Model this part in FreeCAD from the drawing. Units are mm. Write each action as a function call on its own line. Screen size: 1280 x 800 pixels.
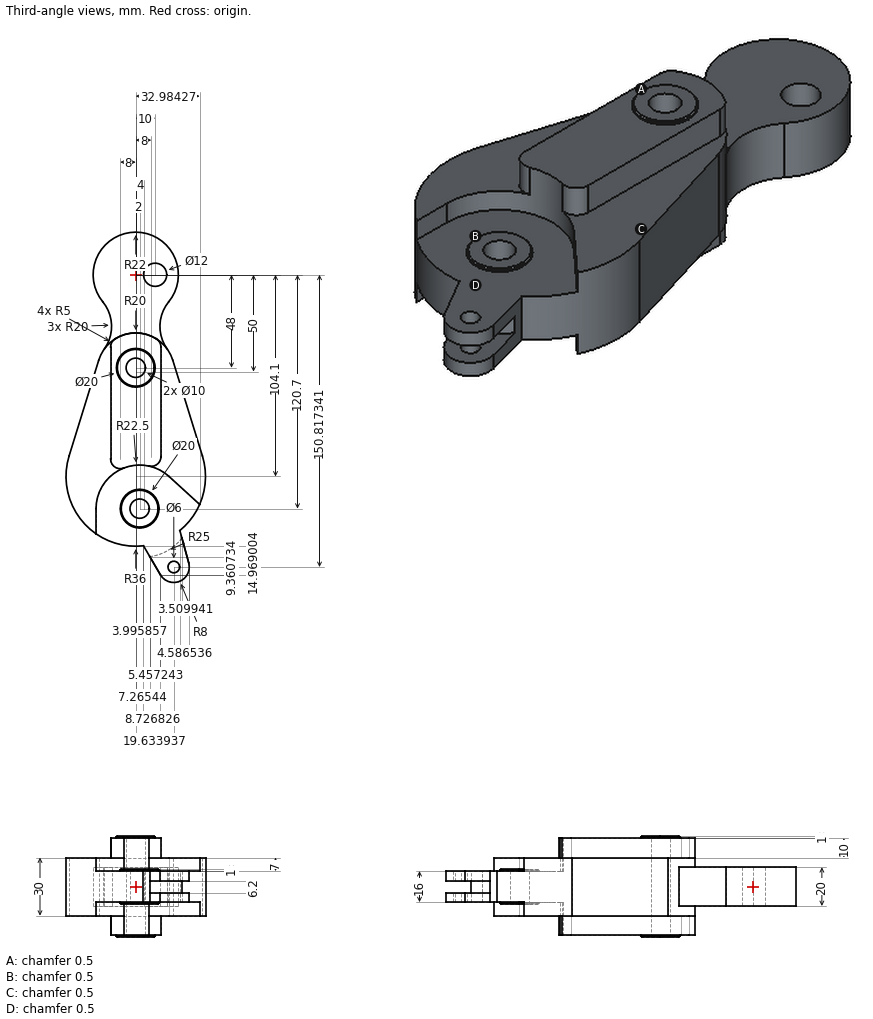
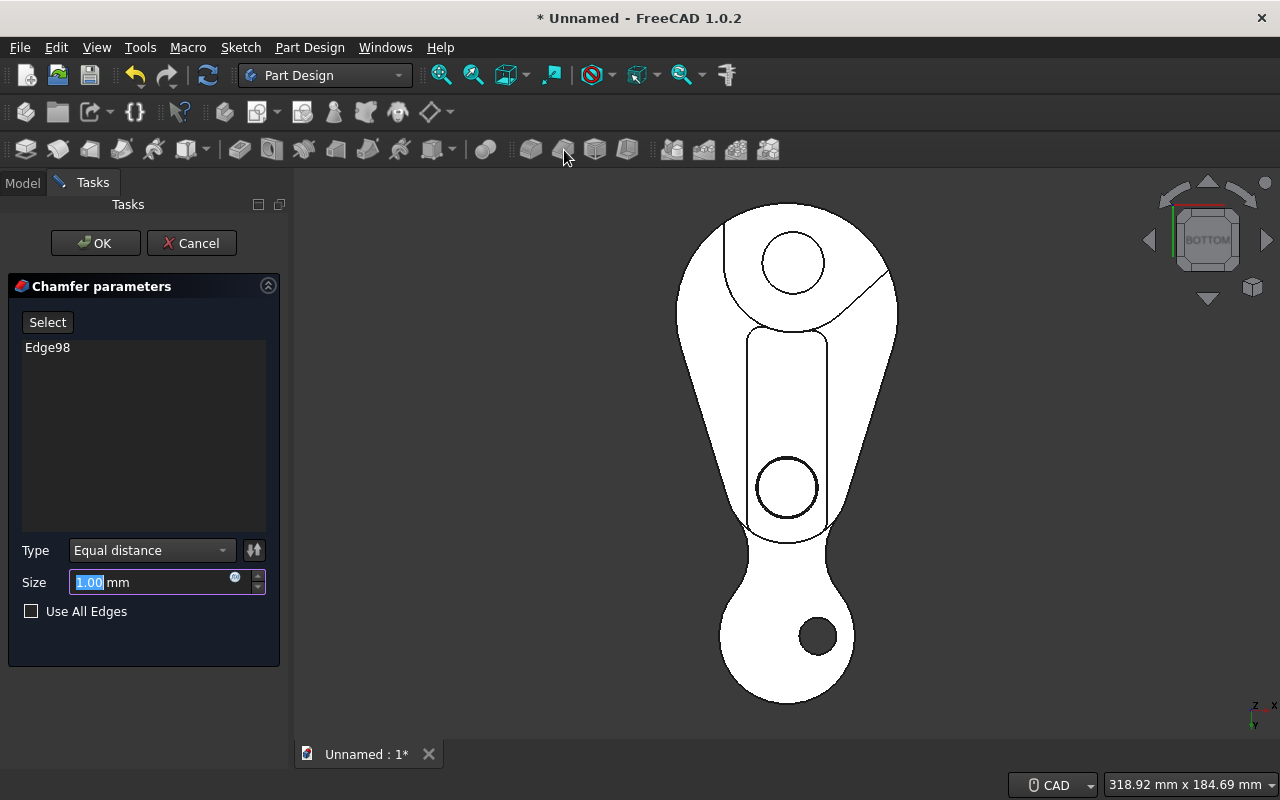
text(0.5)
key(Tab)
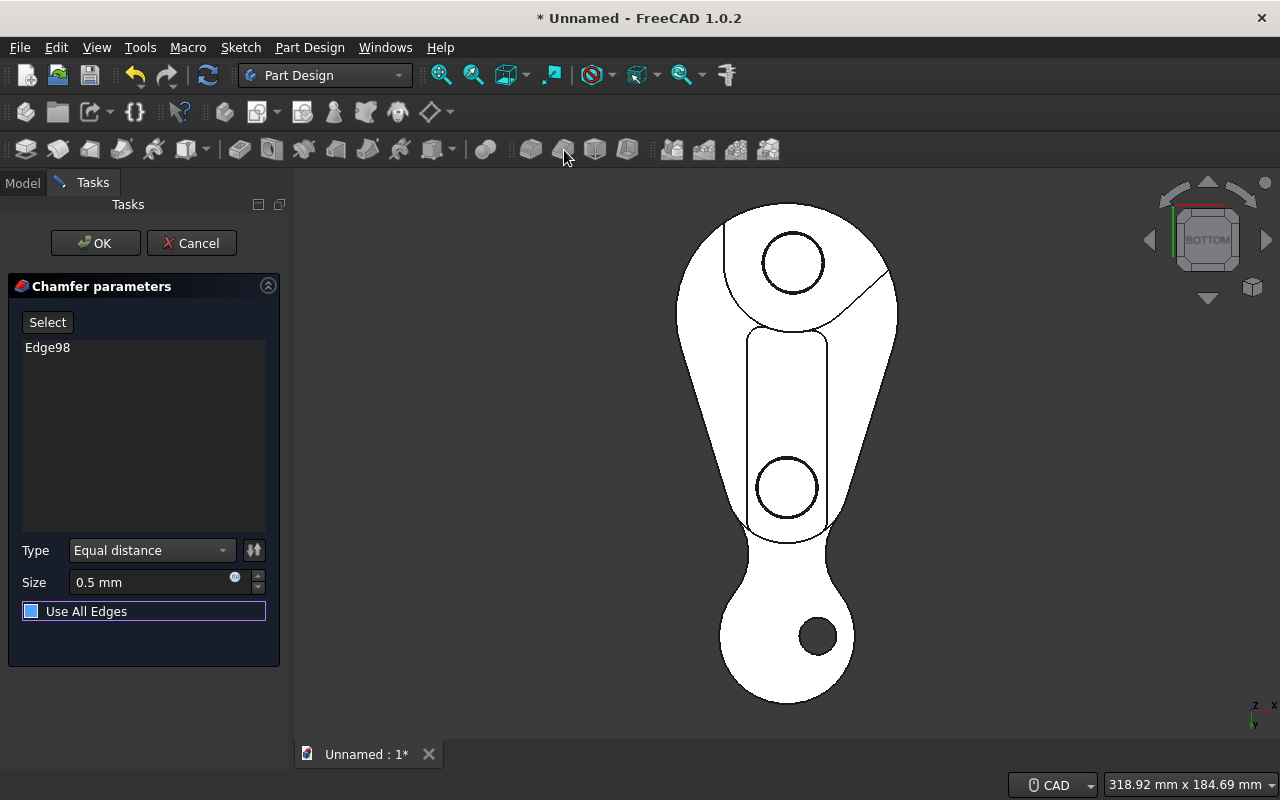
click(96, 243)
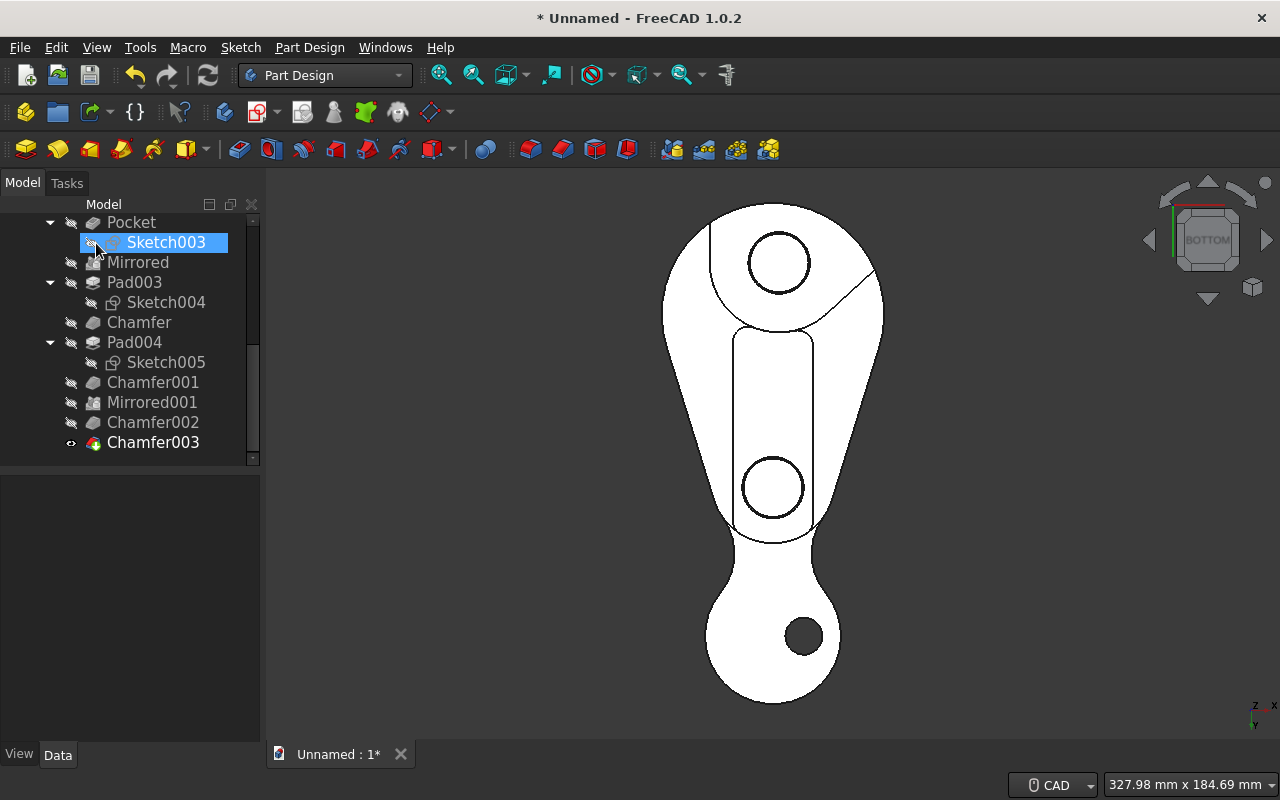
key(0)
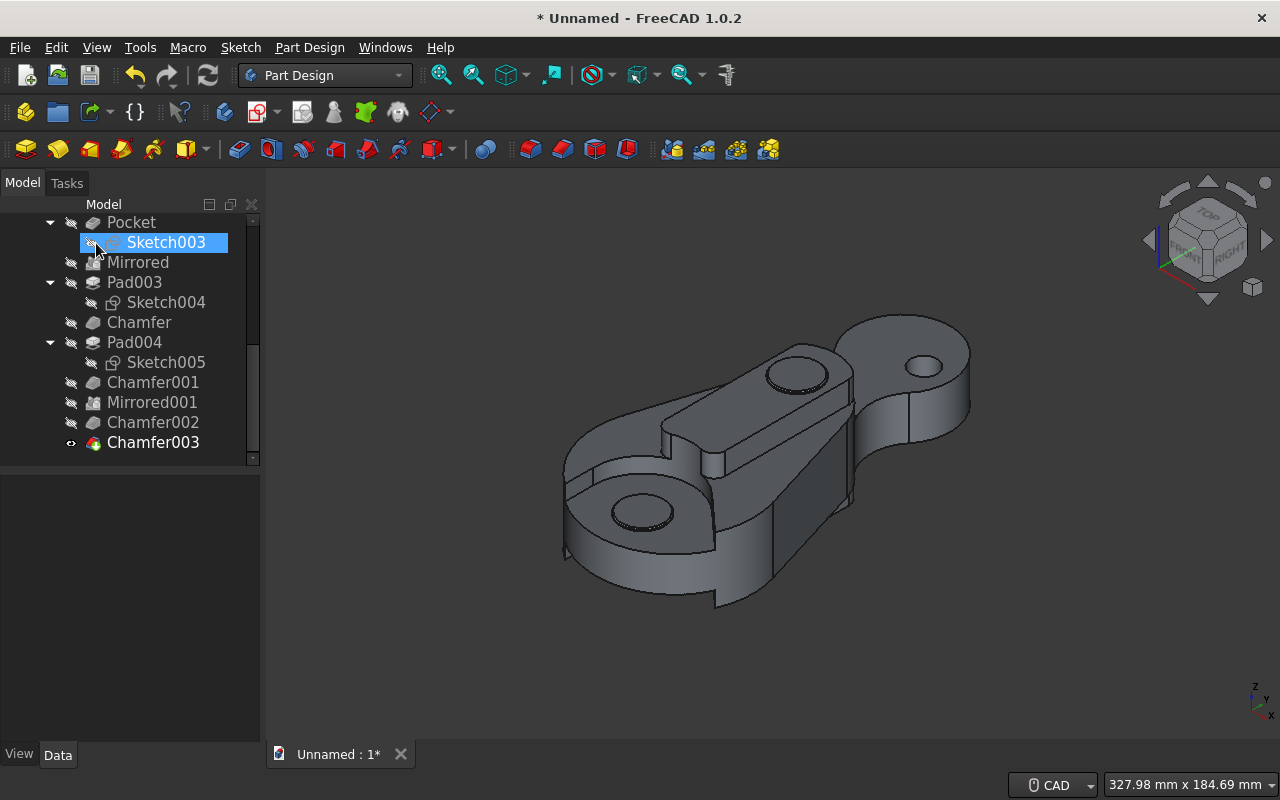
click(797, 373)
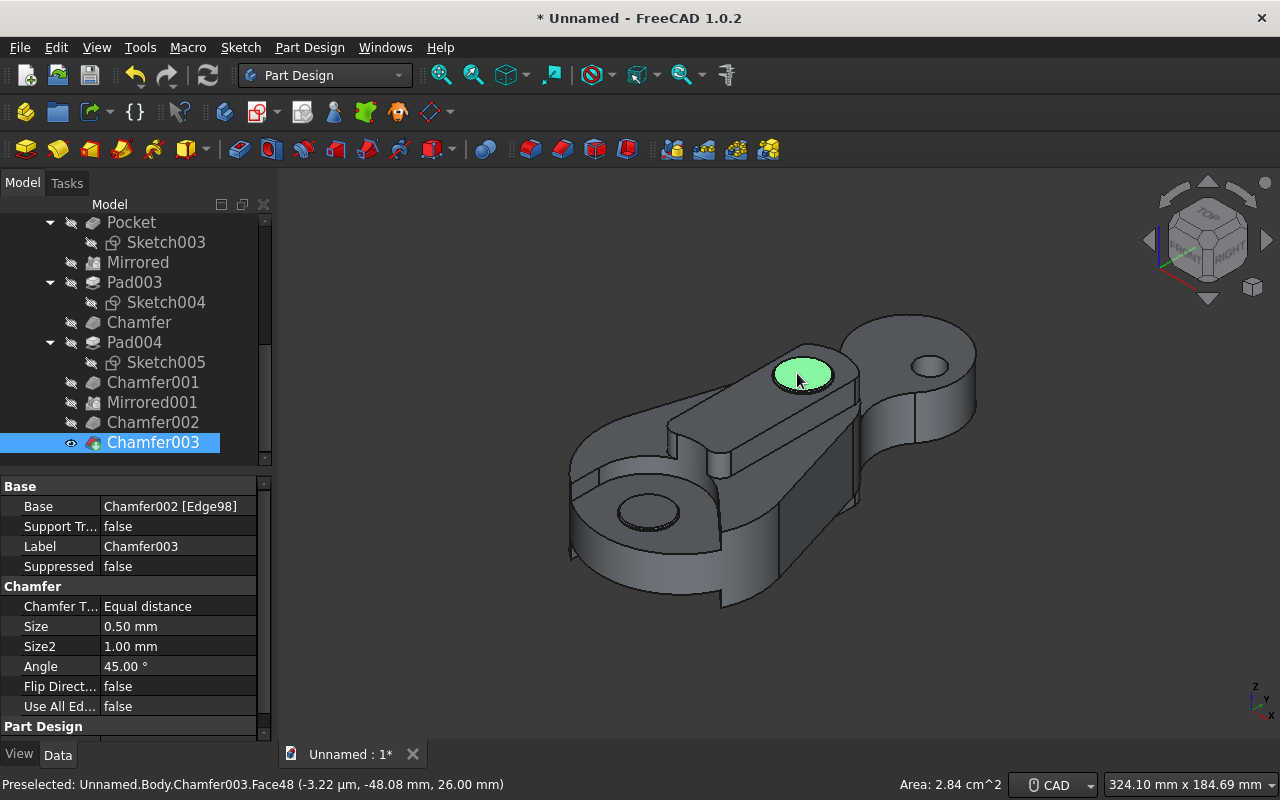
click(258, 112)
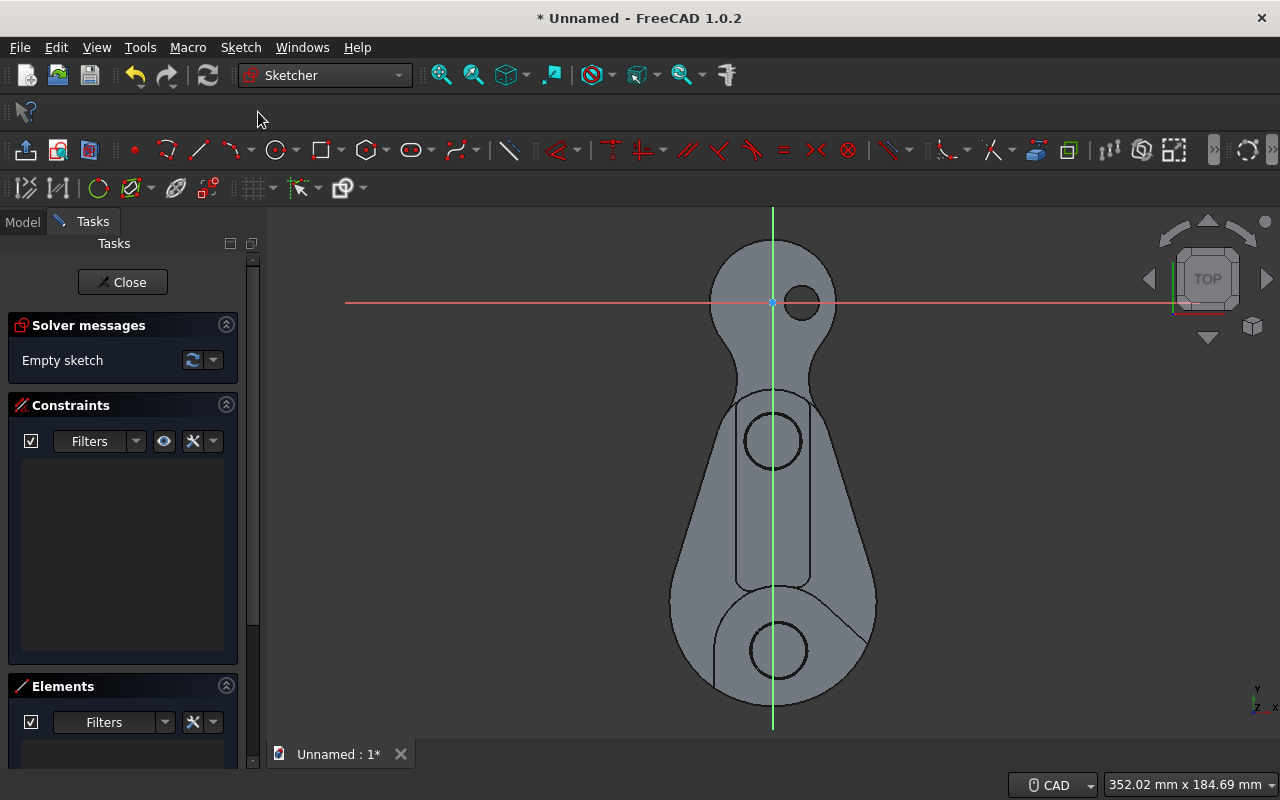
click(276, 150)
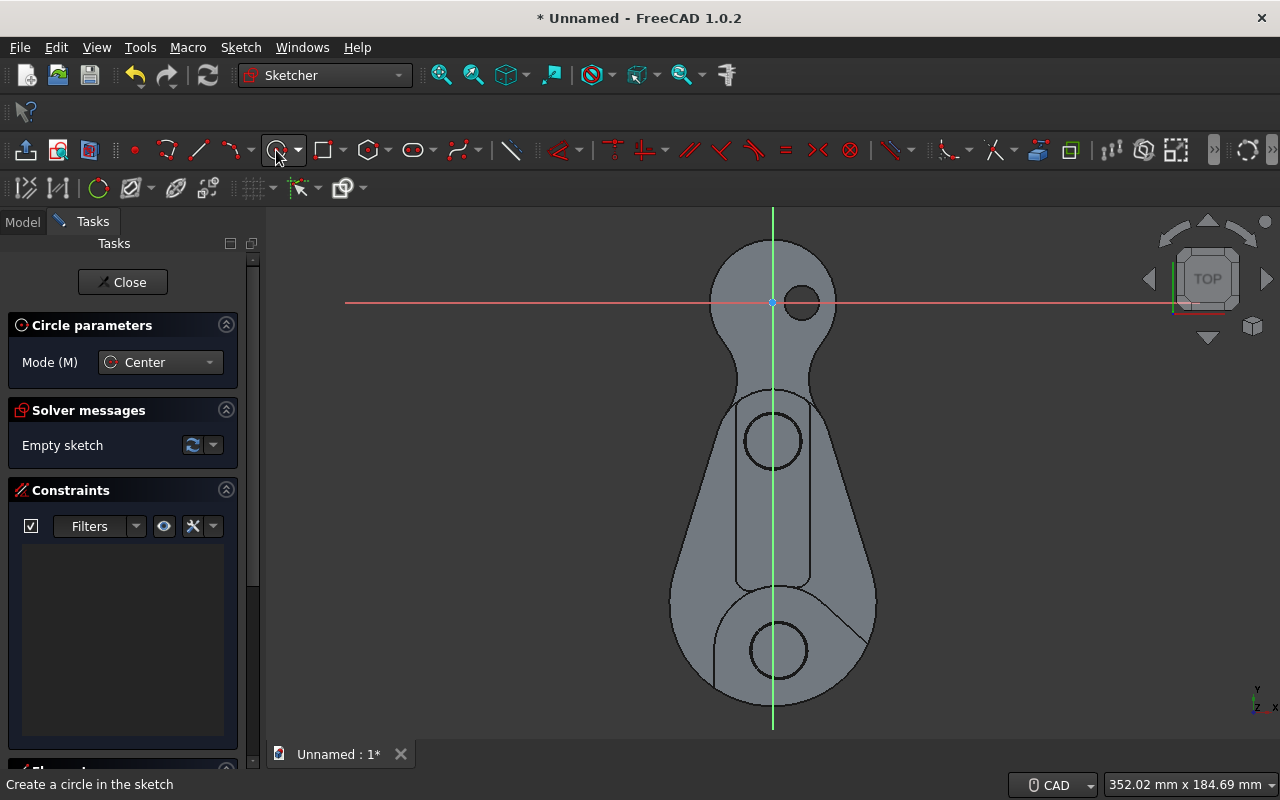
scroll(773, 441, up, 3)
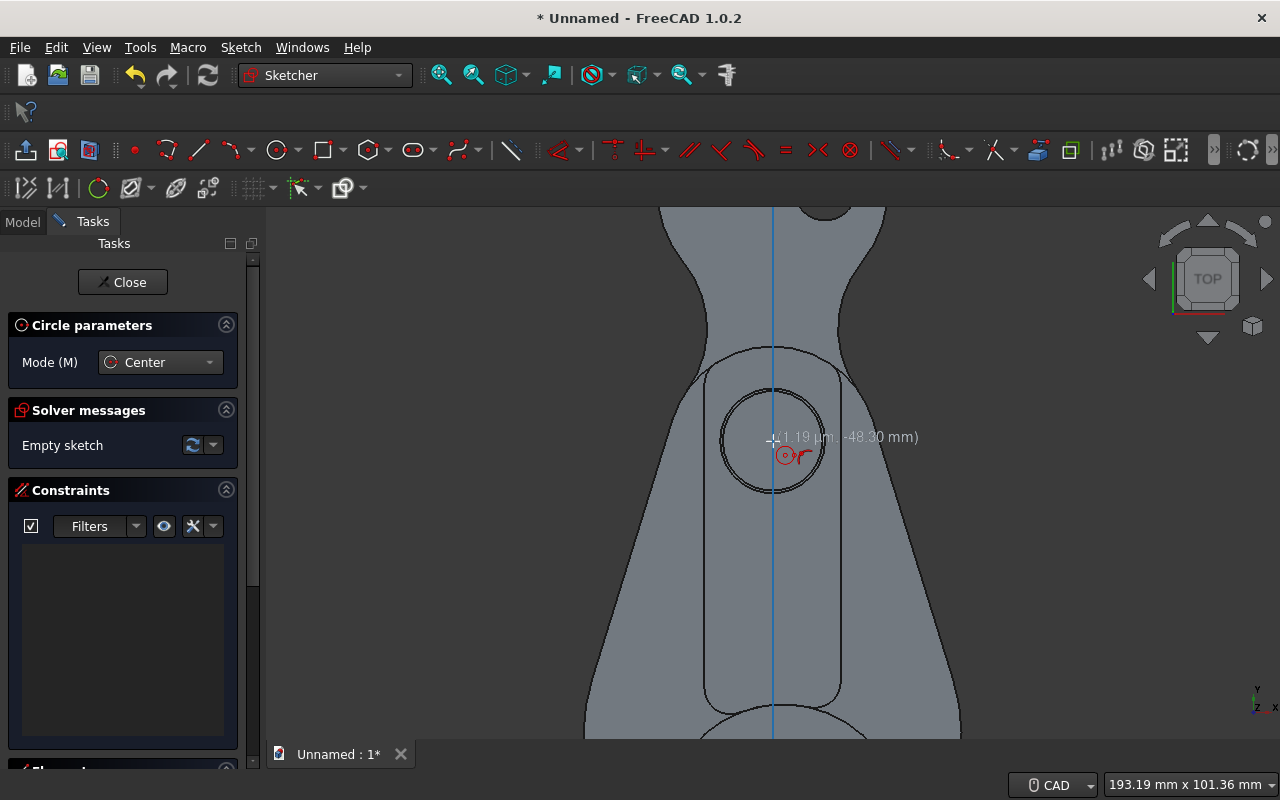
click(773, 441)
click(791, 422)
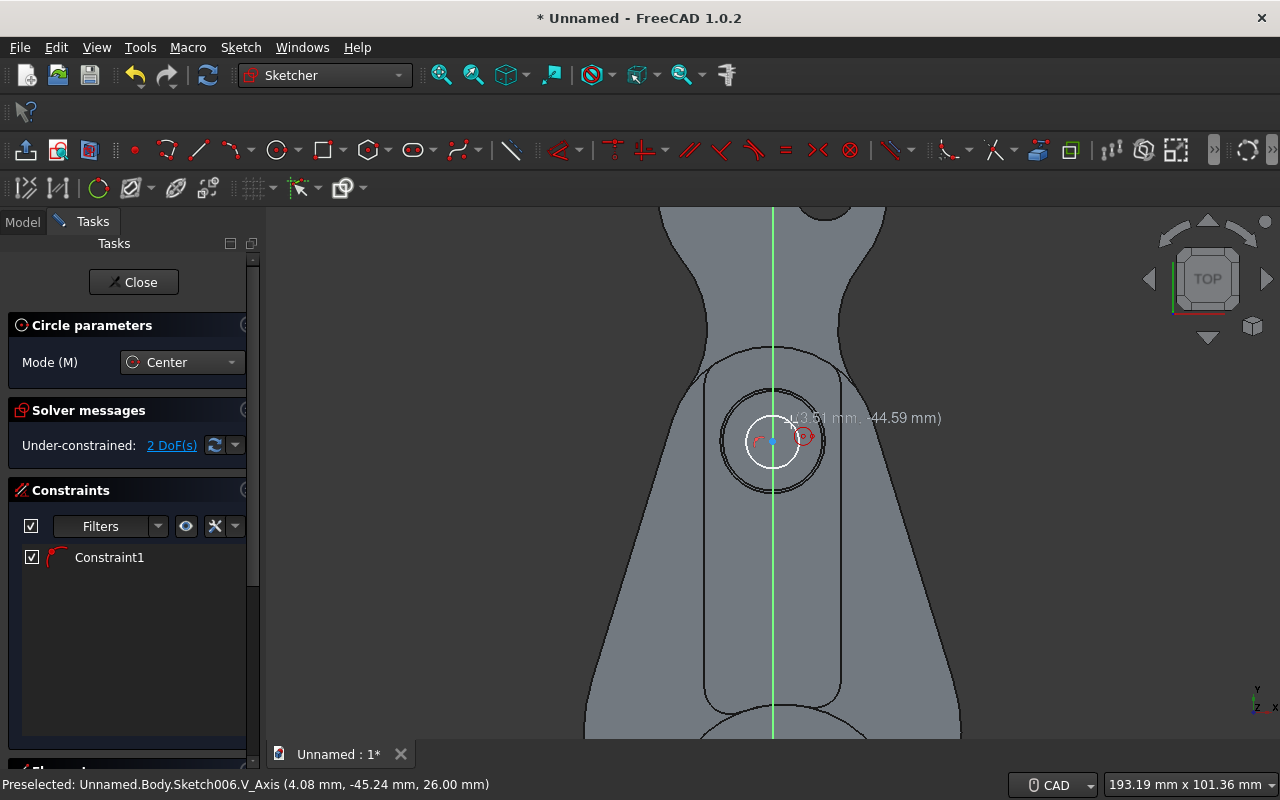
scroll(615, 417, down, 3)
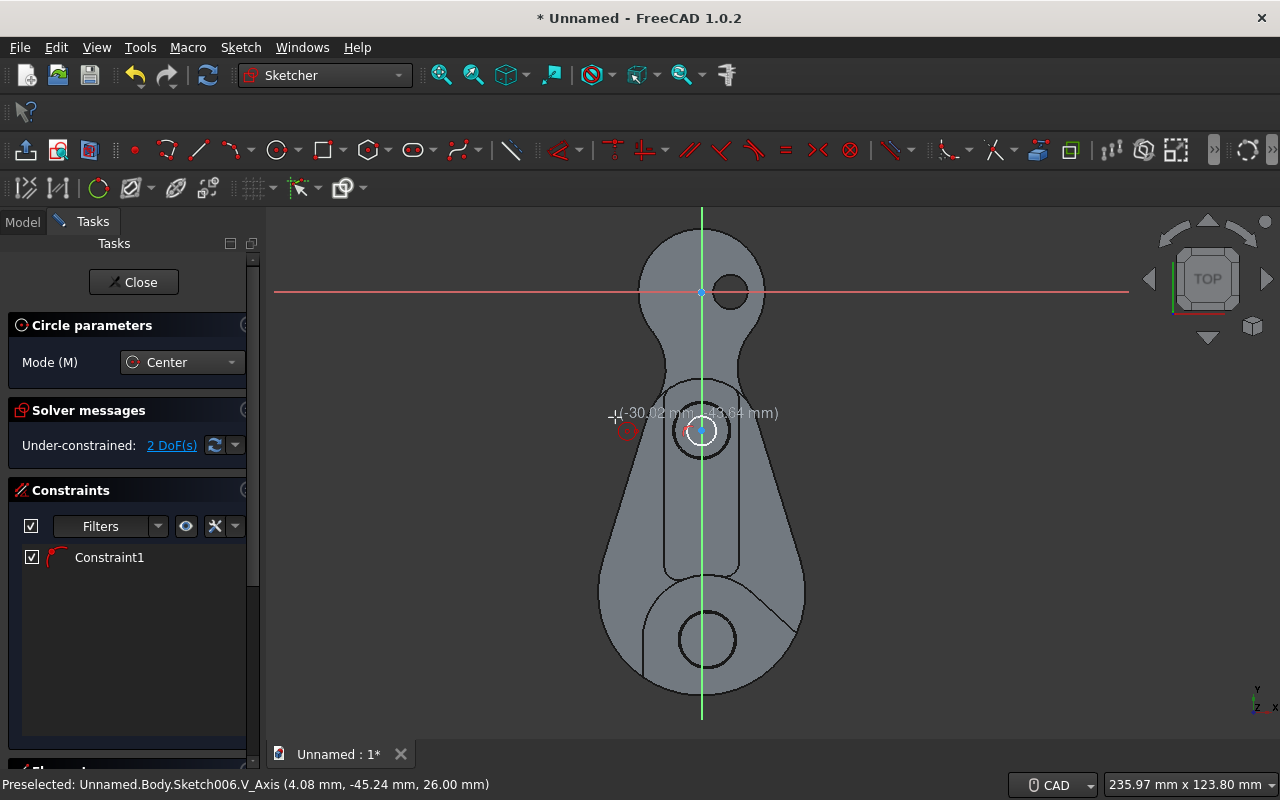
scroll(707, 640, up, 6)